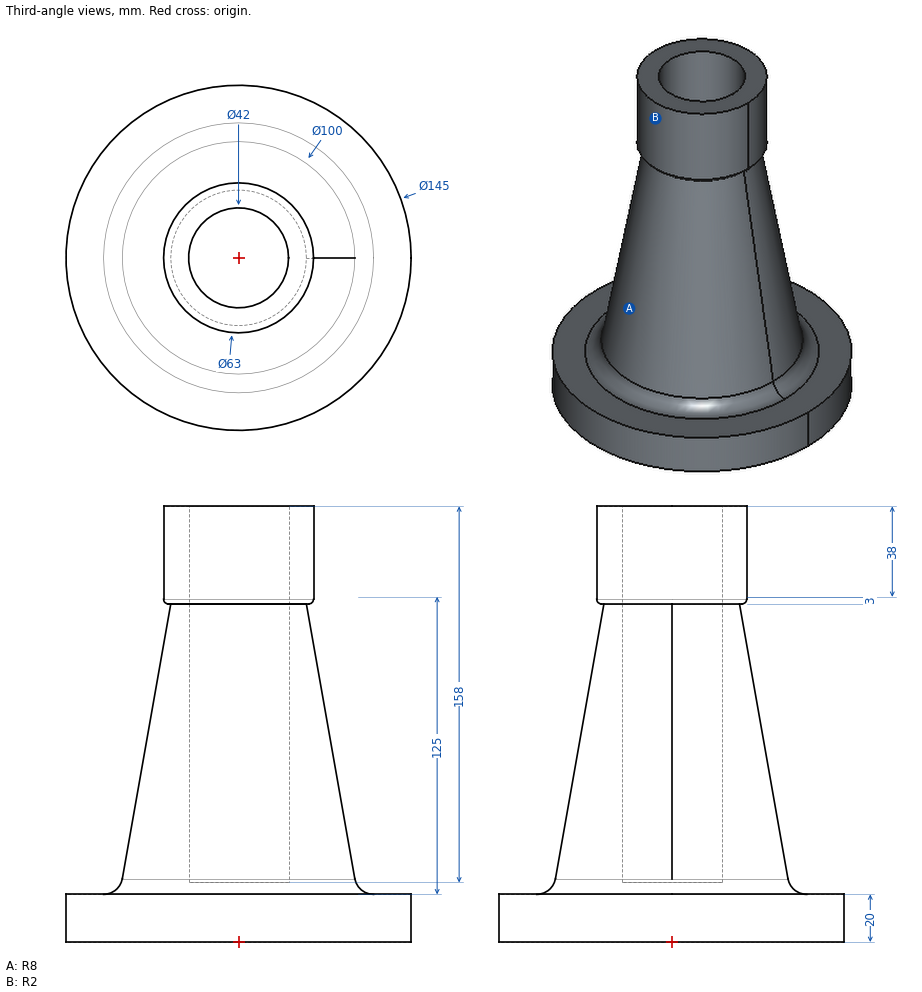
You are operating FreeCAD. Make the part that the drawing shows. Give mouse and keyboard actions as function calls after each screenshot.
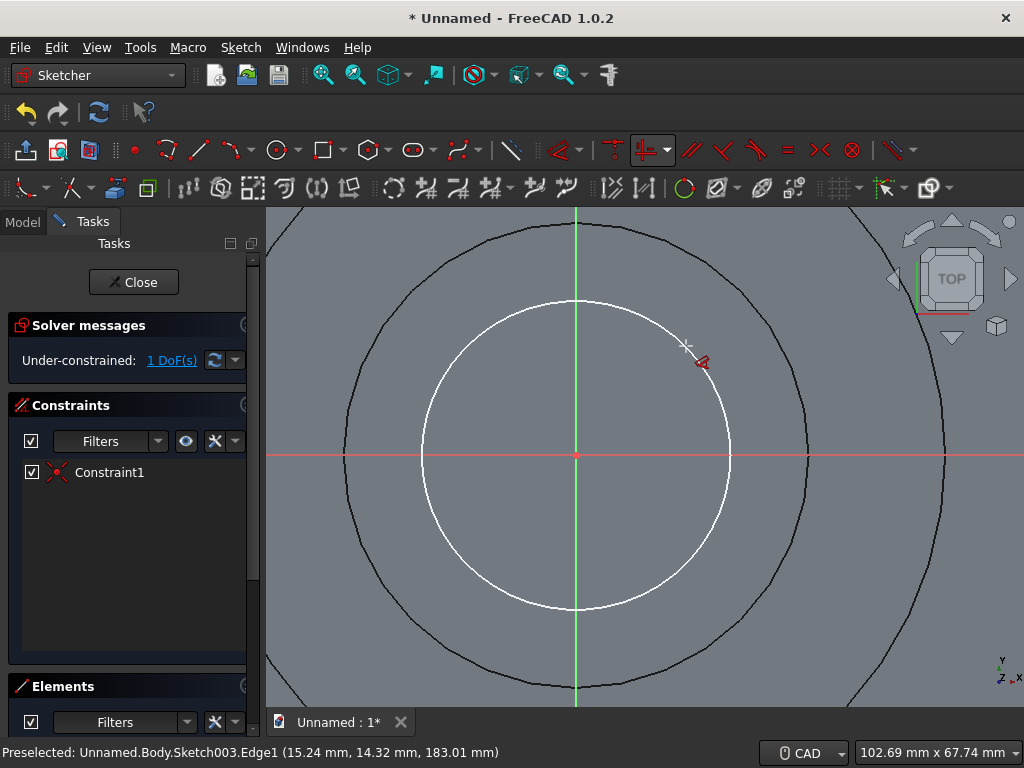
click(685, 346)
click(708, 323)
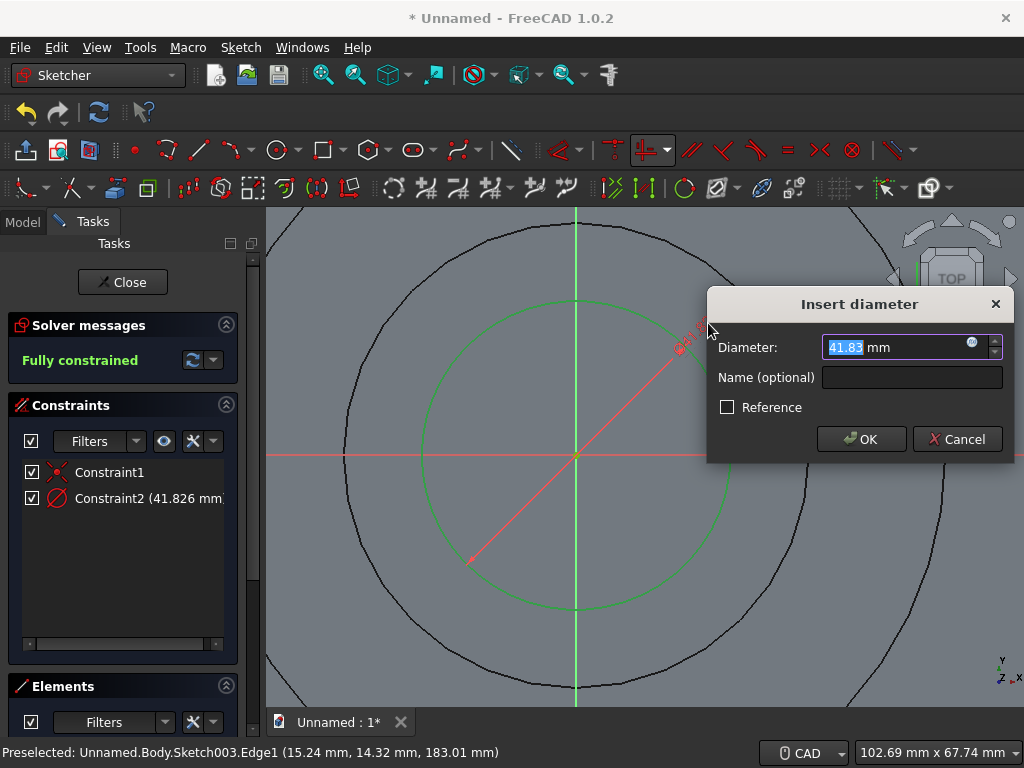
text(42)
key(Return)
key(Escape)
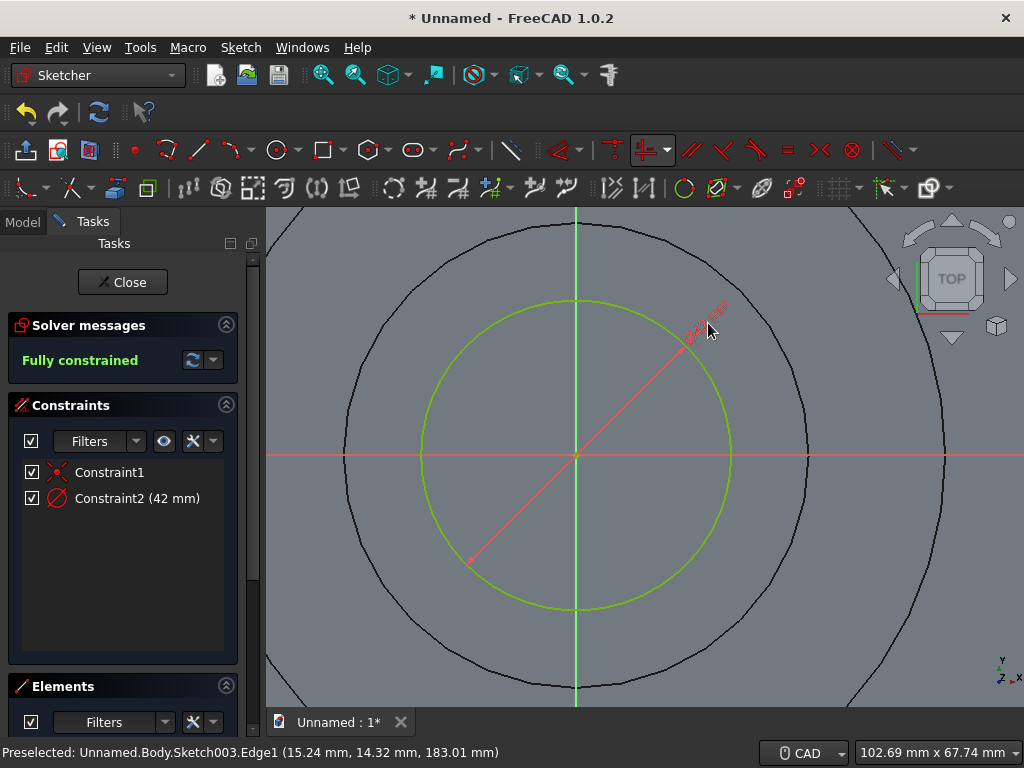
click(123, 282)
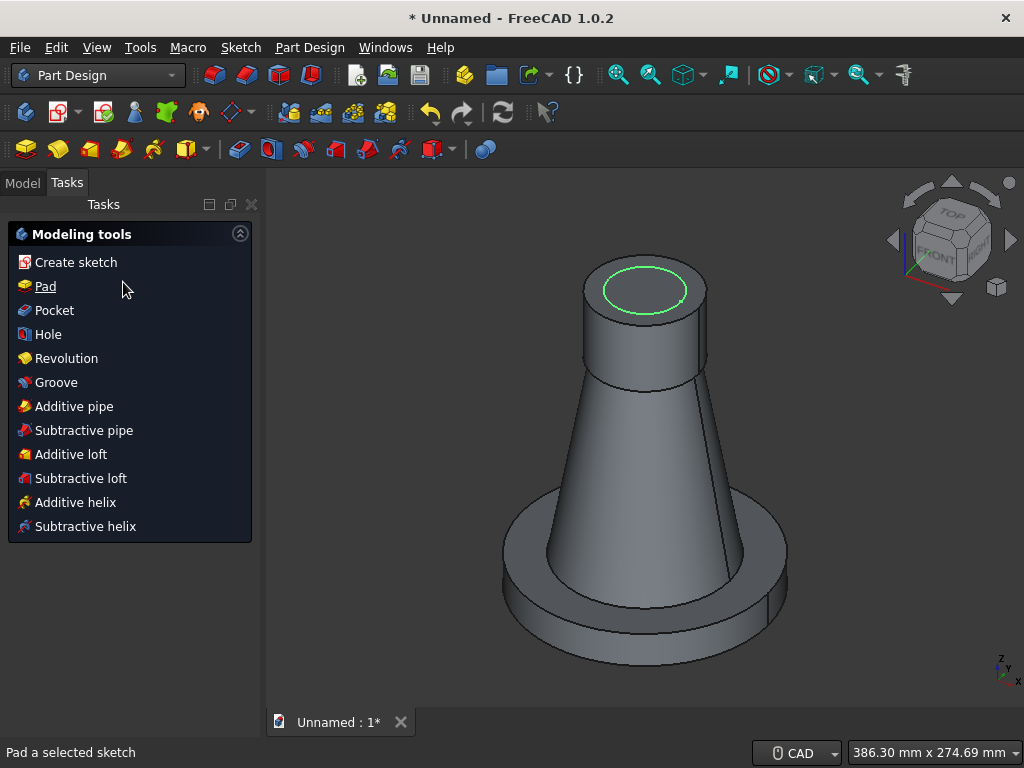
click(240, 150)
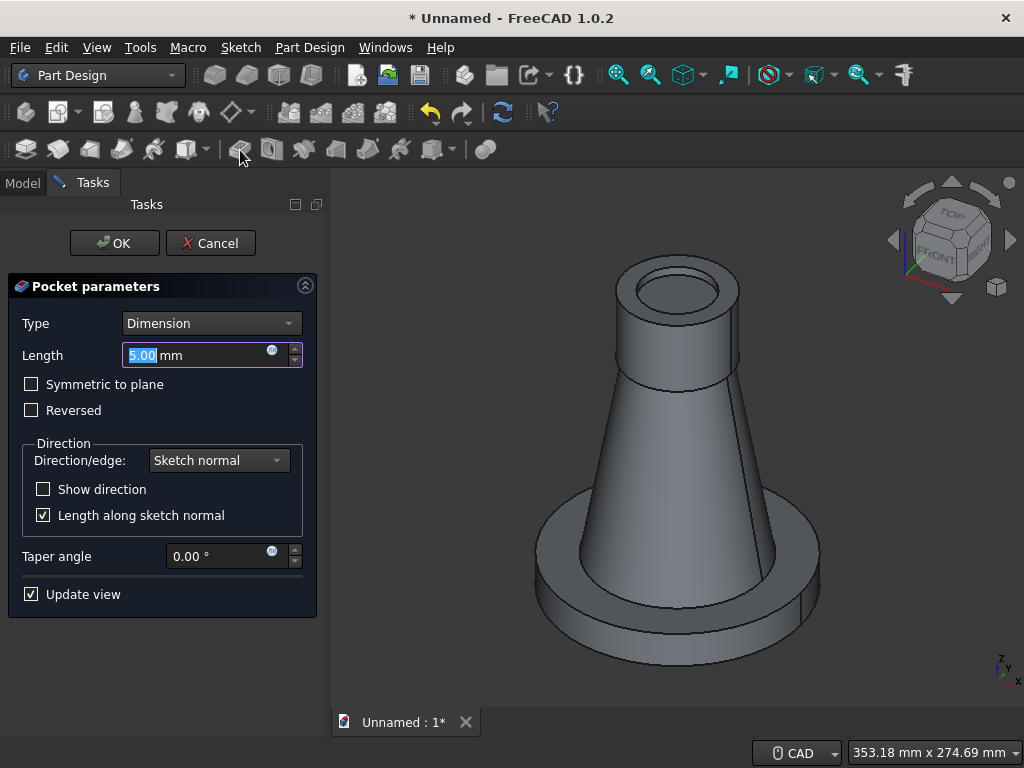
text(158)
key(Tab)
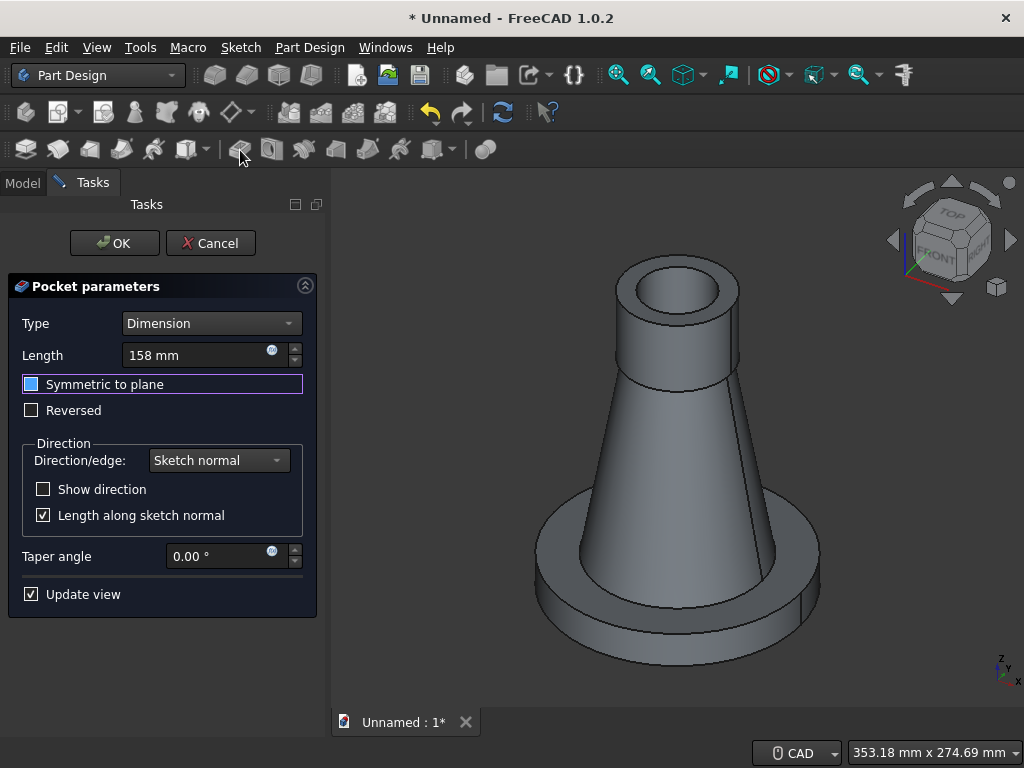
click(115, 243)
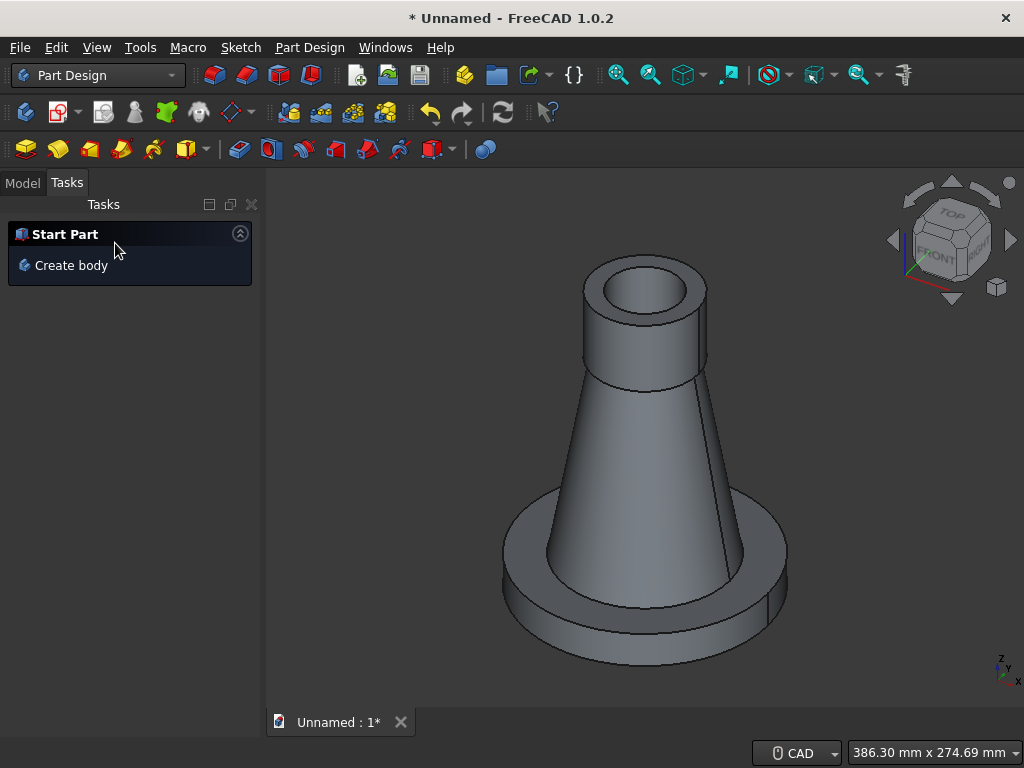
key(0)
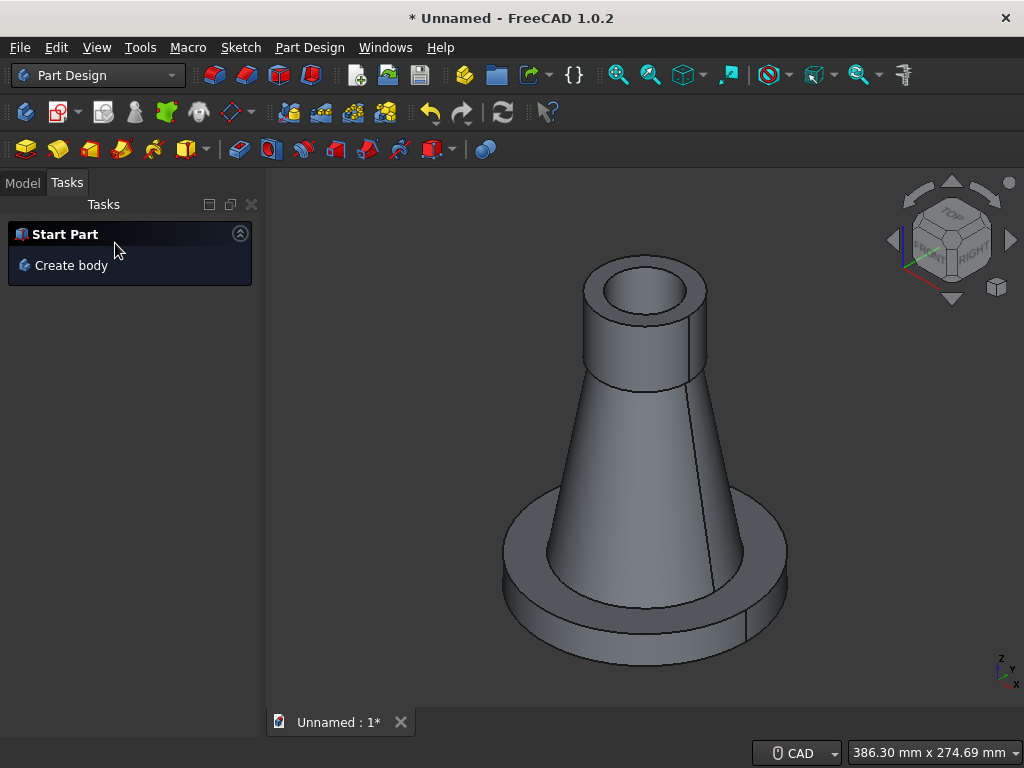
key(2)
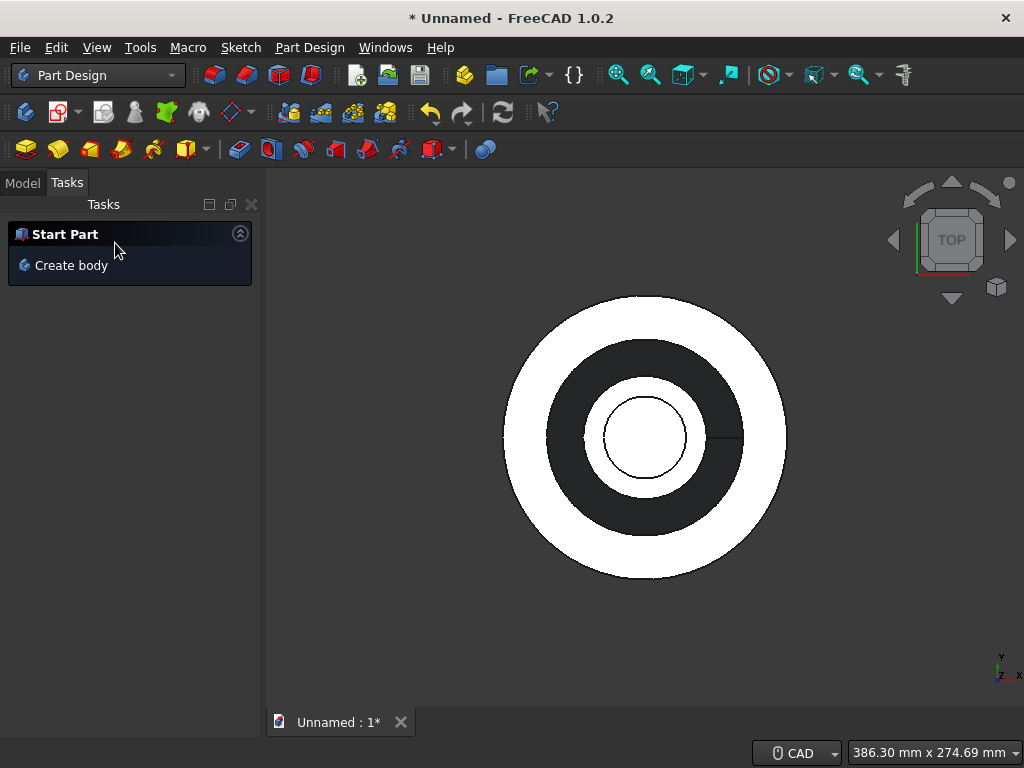
key(1)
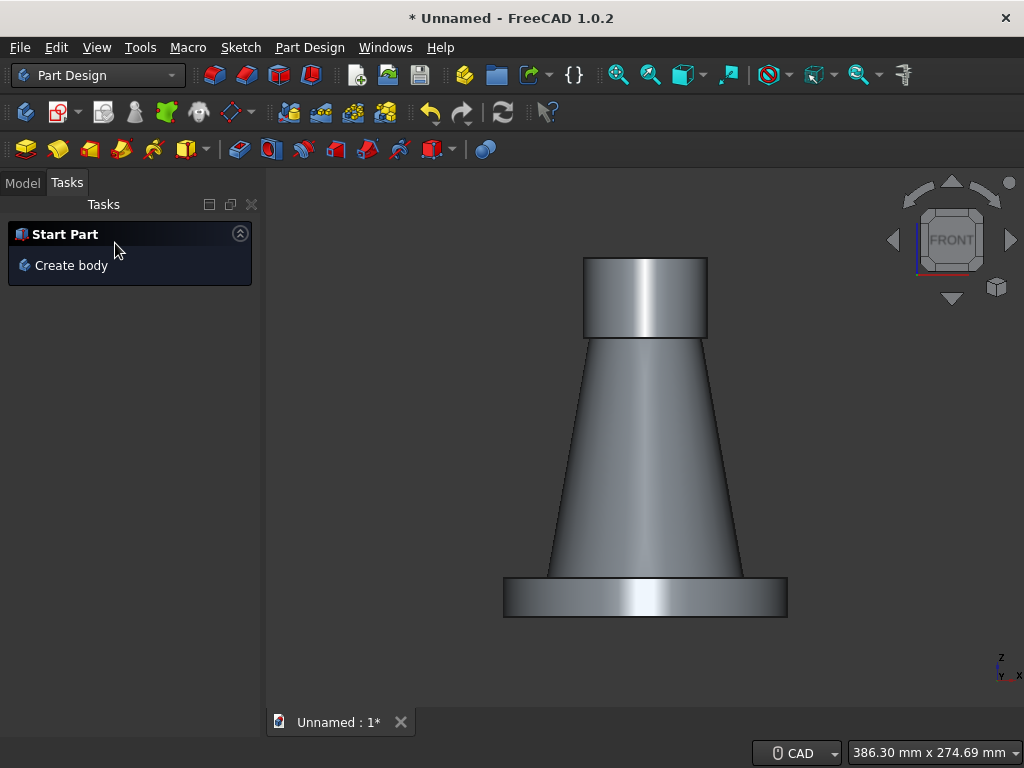
key(3)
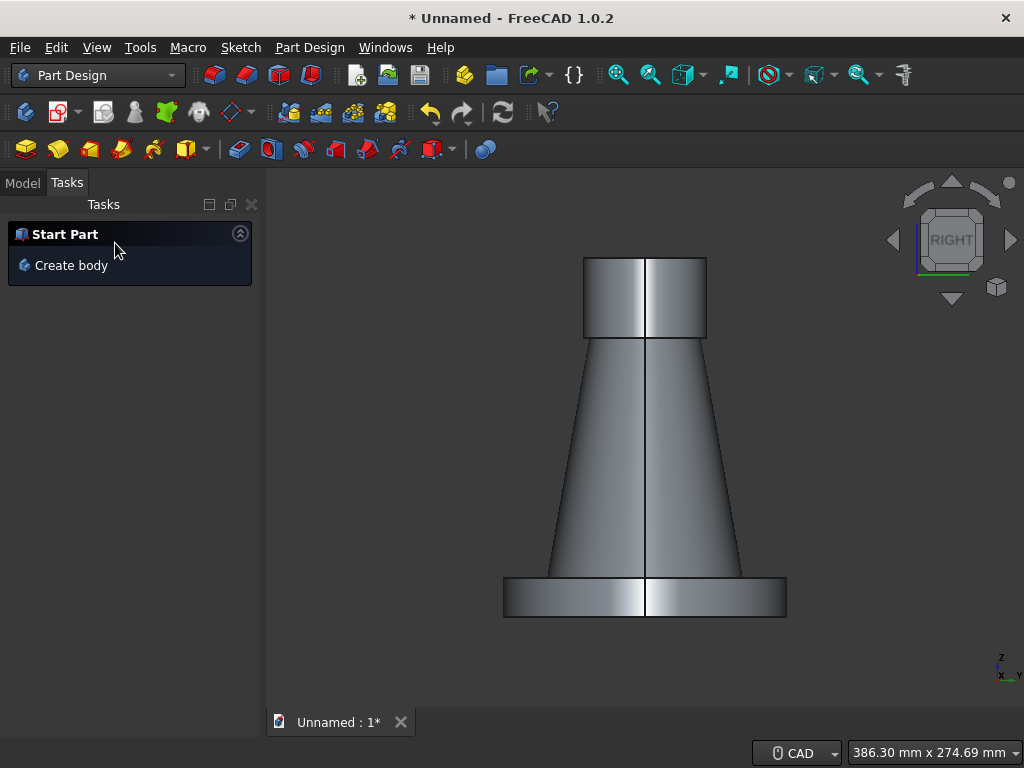
key(5)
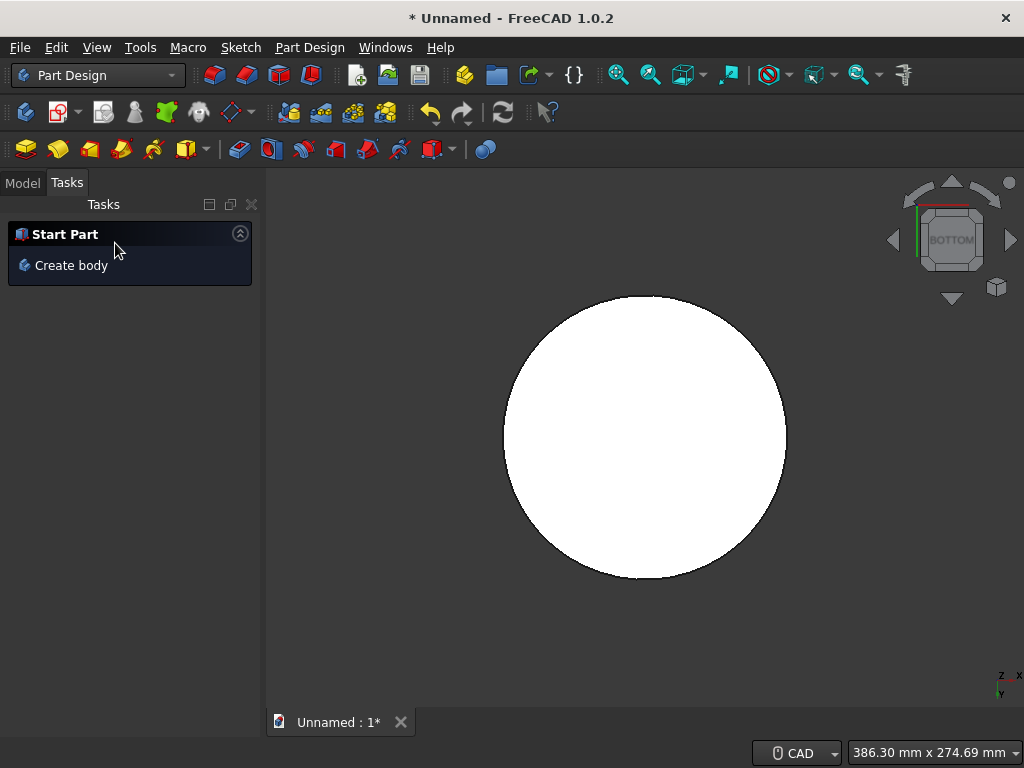
key(4)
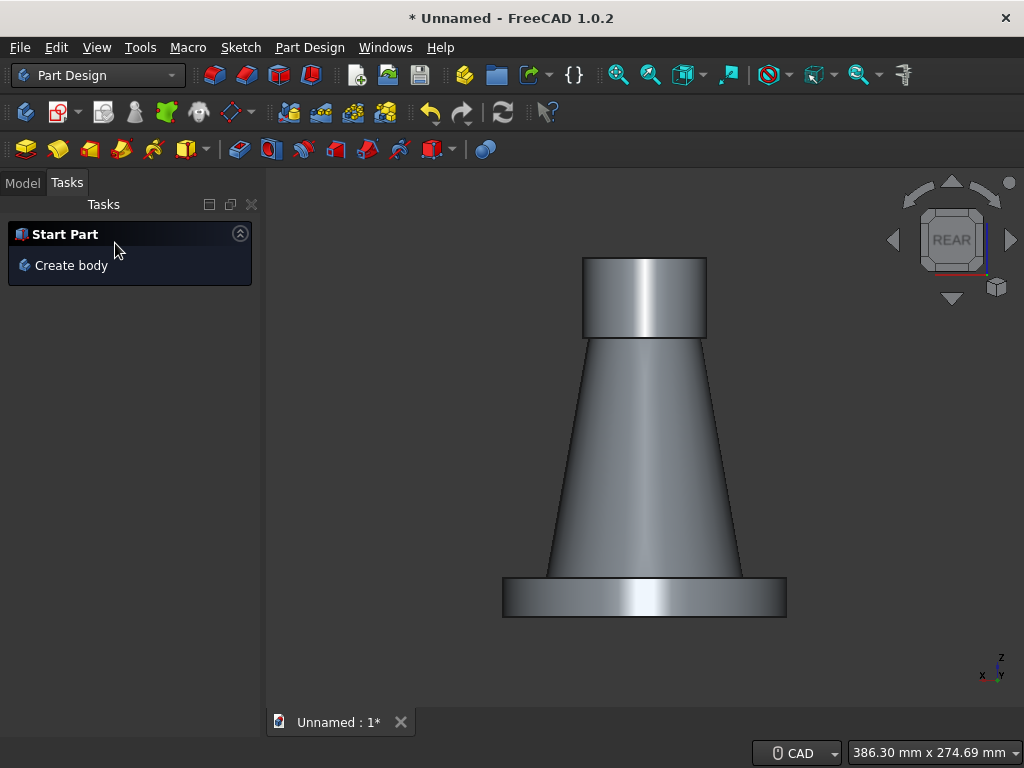
key(6)